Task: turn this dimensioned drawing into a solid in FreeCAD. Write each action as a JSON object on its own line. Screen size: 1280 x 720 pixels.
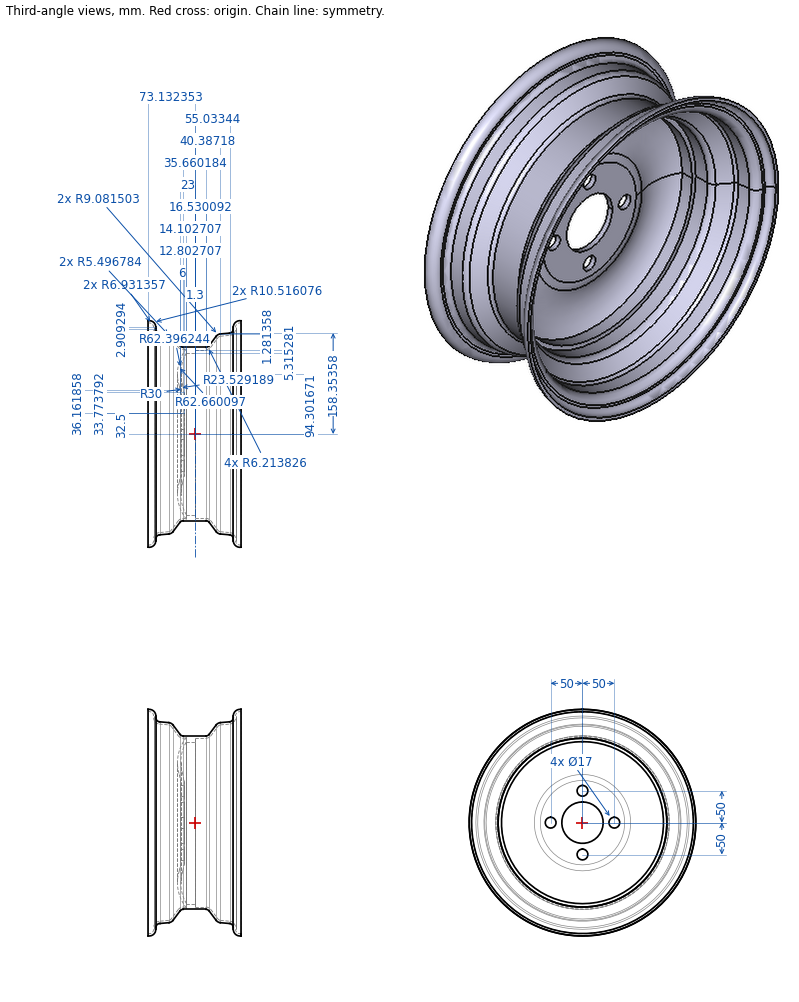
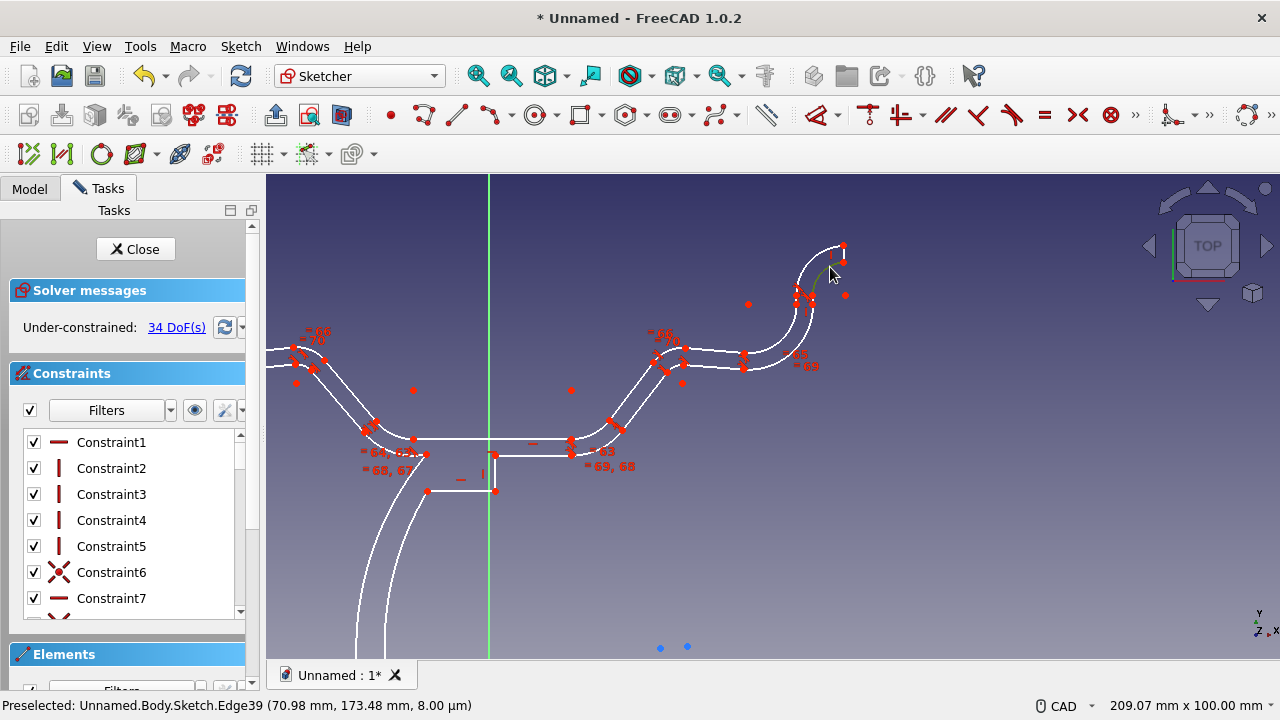
{"action": "key", "text": "e"}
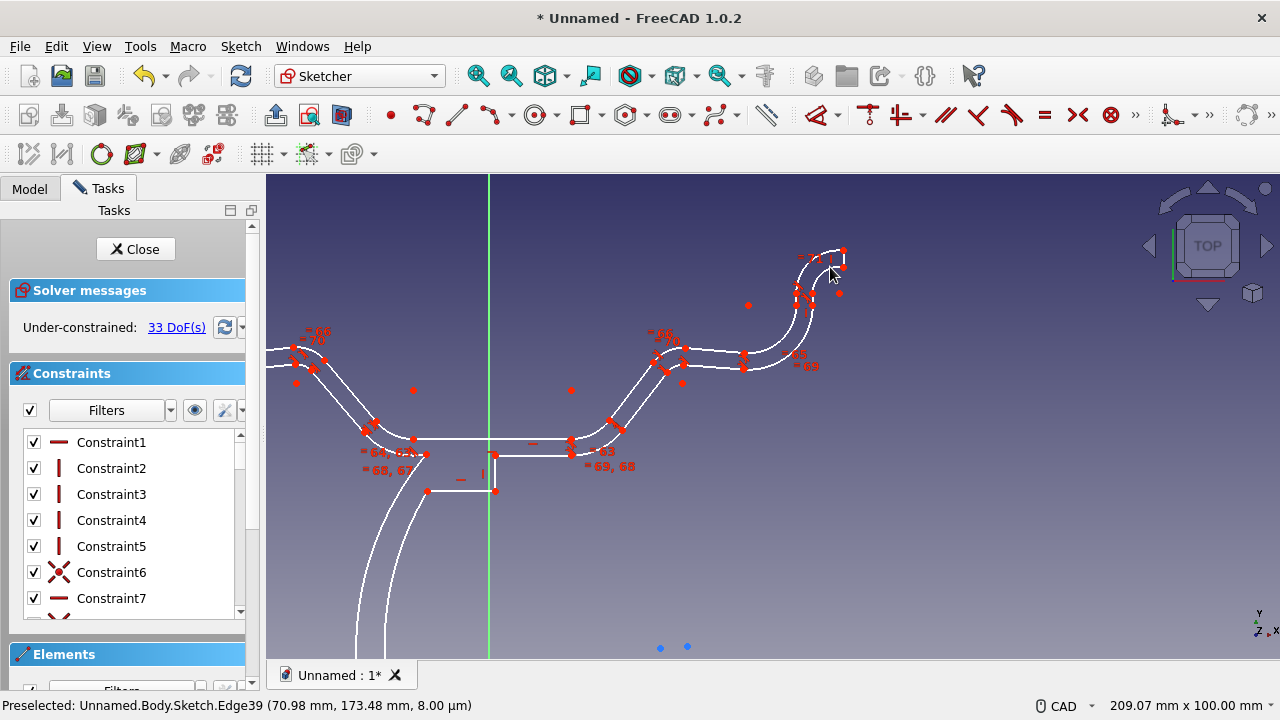
{"action": "left_click", "coordinate": [682, 384]}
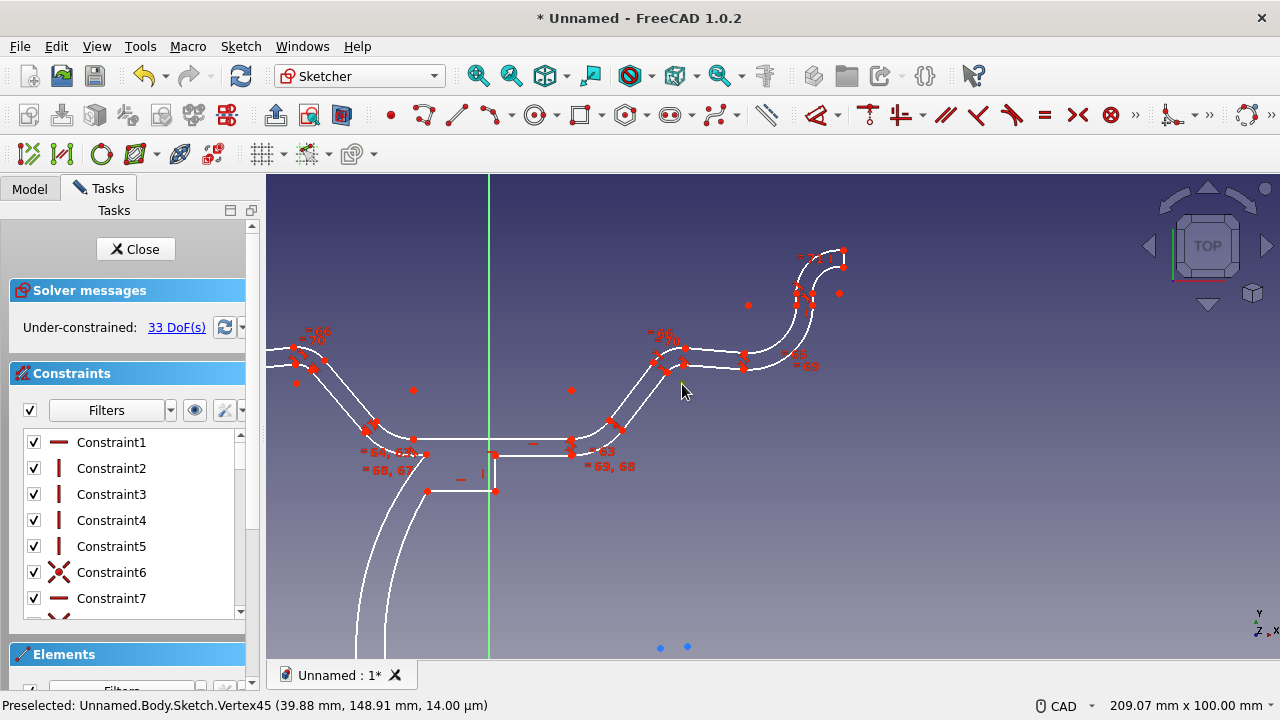
{"action": "left_click", "coordinate": [297, 383]}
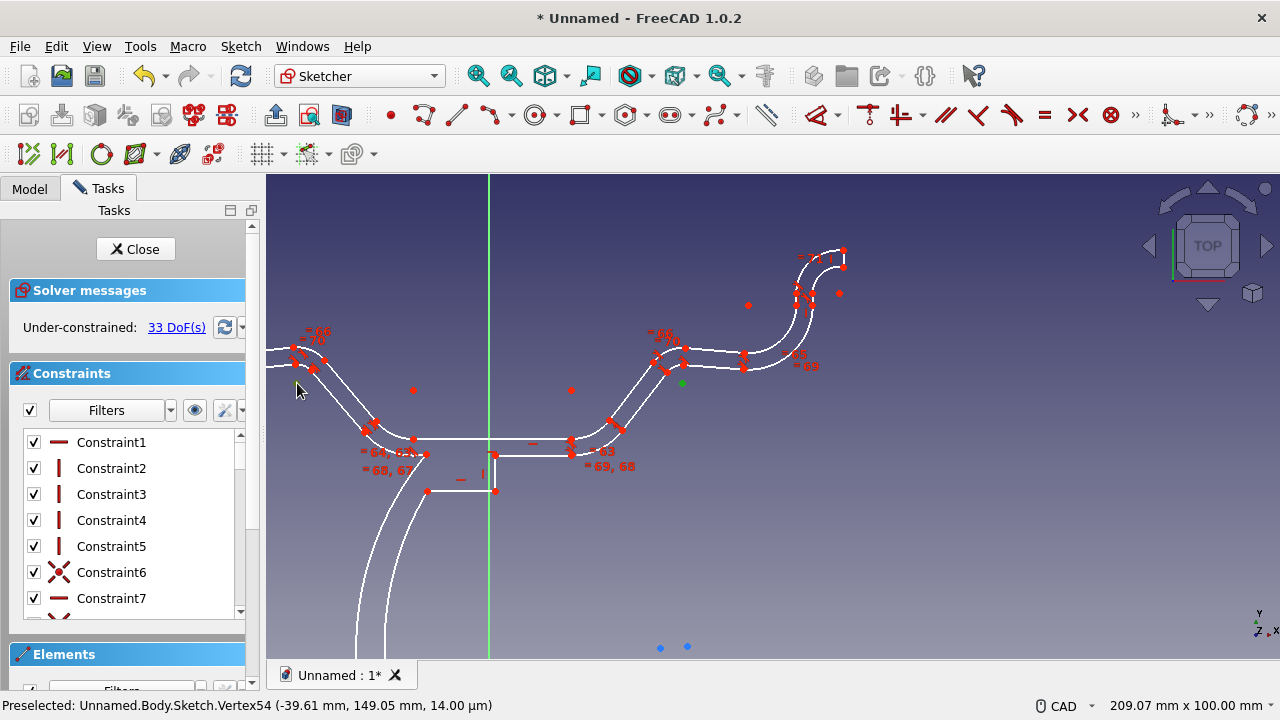
{"action": "left_click", "coordinate": [489, 600]}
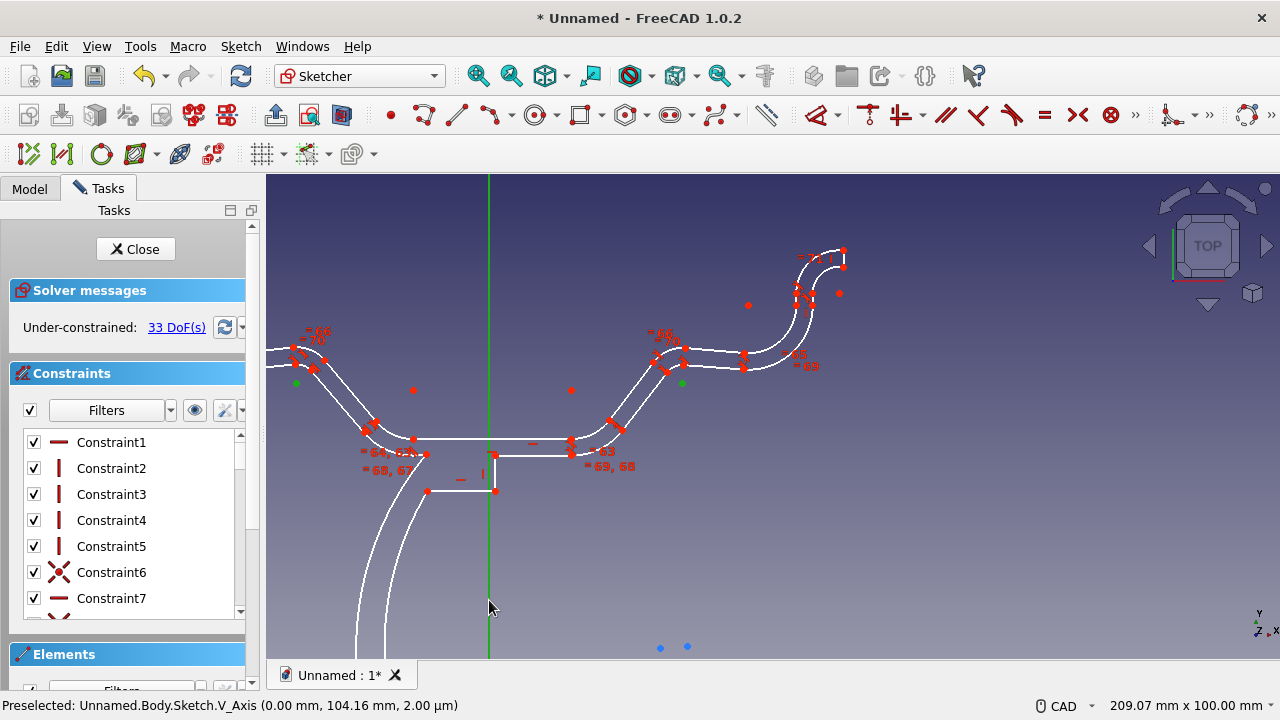
{"action": "left_click", "coordinate": [1078, 116]}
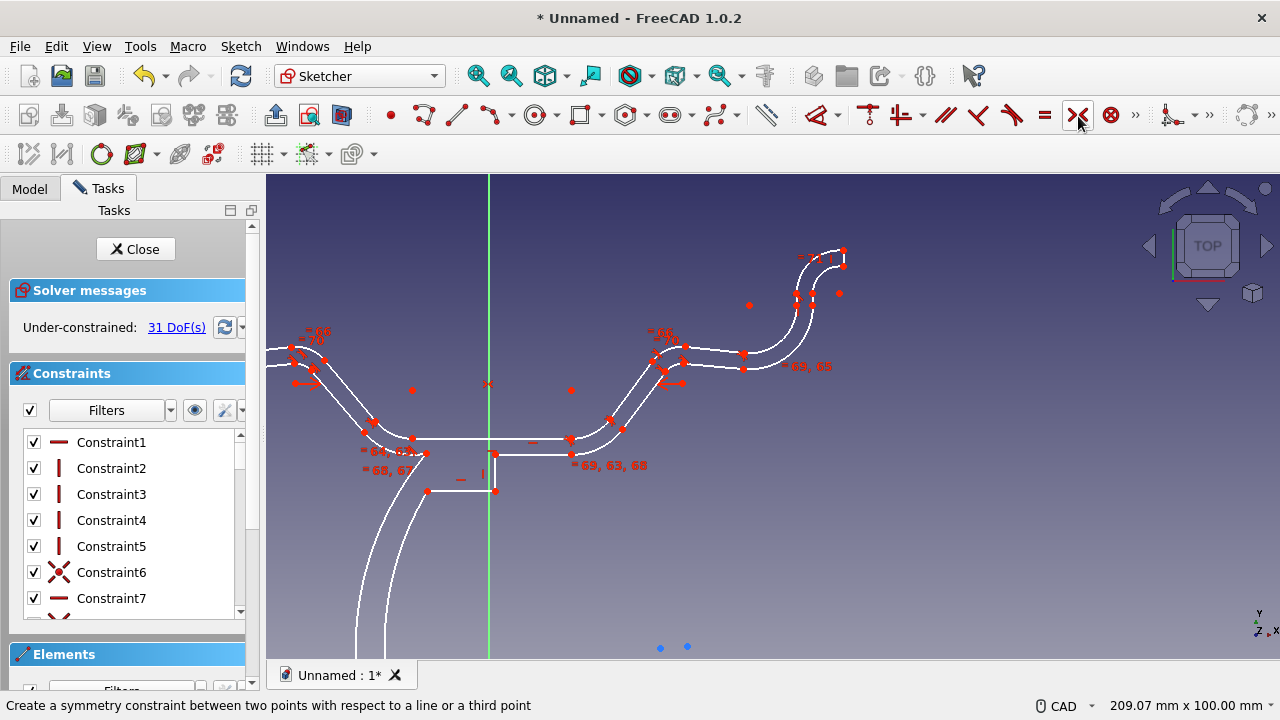
{"action": "scroll", "coordinate": [830, 266], "scroll_direction": "down", "scroll_amount": 5}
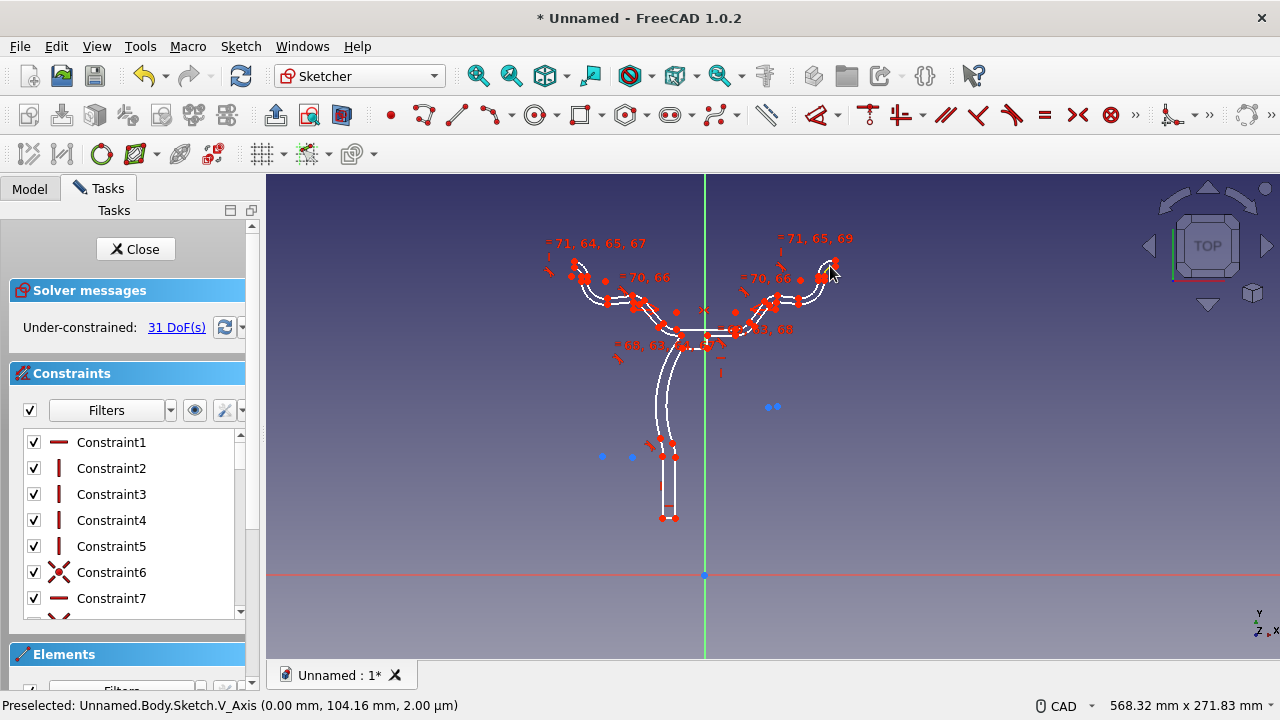
{"action": "left_click", "coordinate": [605, 281]}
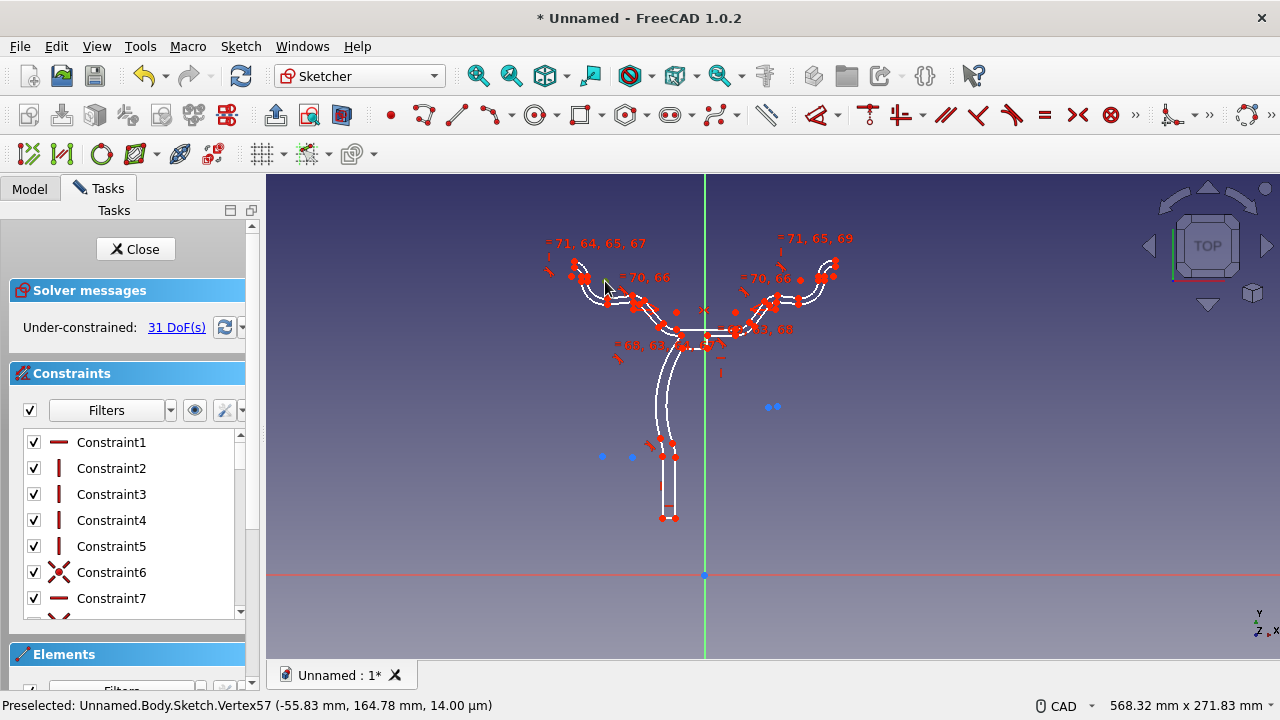
{"action": "left_click", "coordinate": [801, 281]}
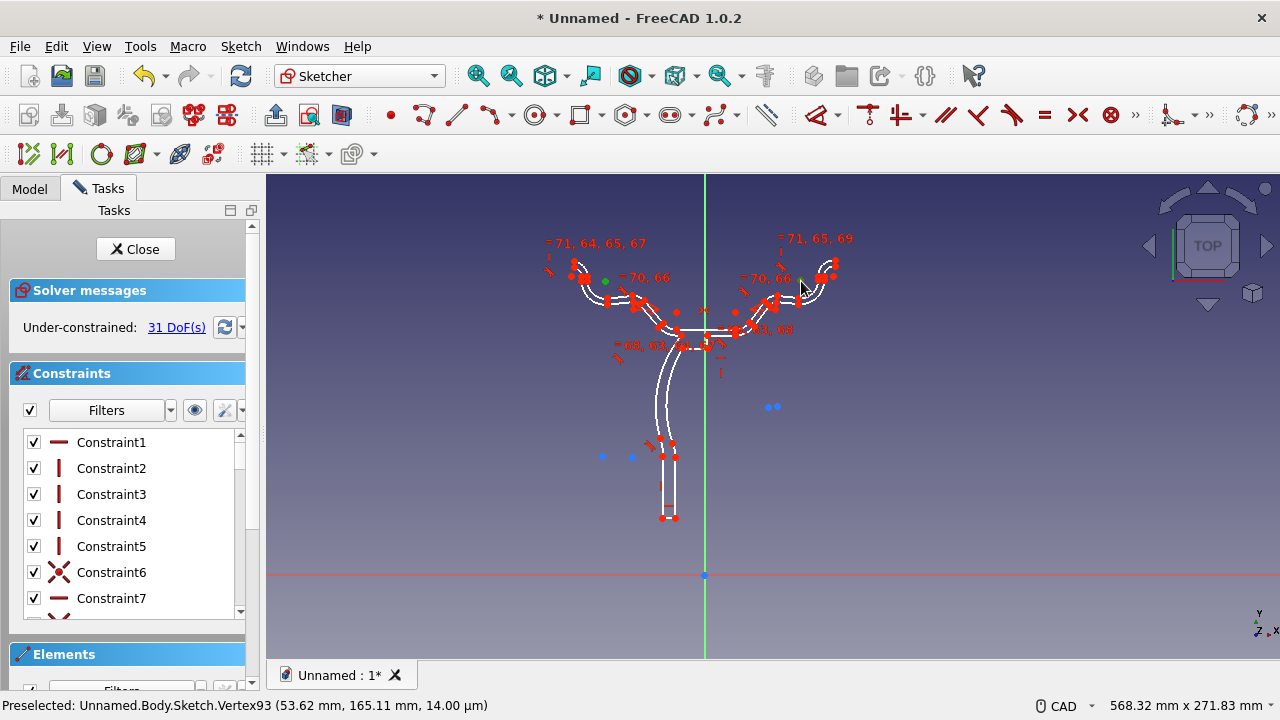
{"action": "left_click", "coordinate": [705, 539]}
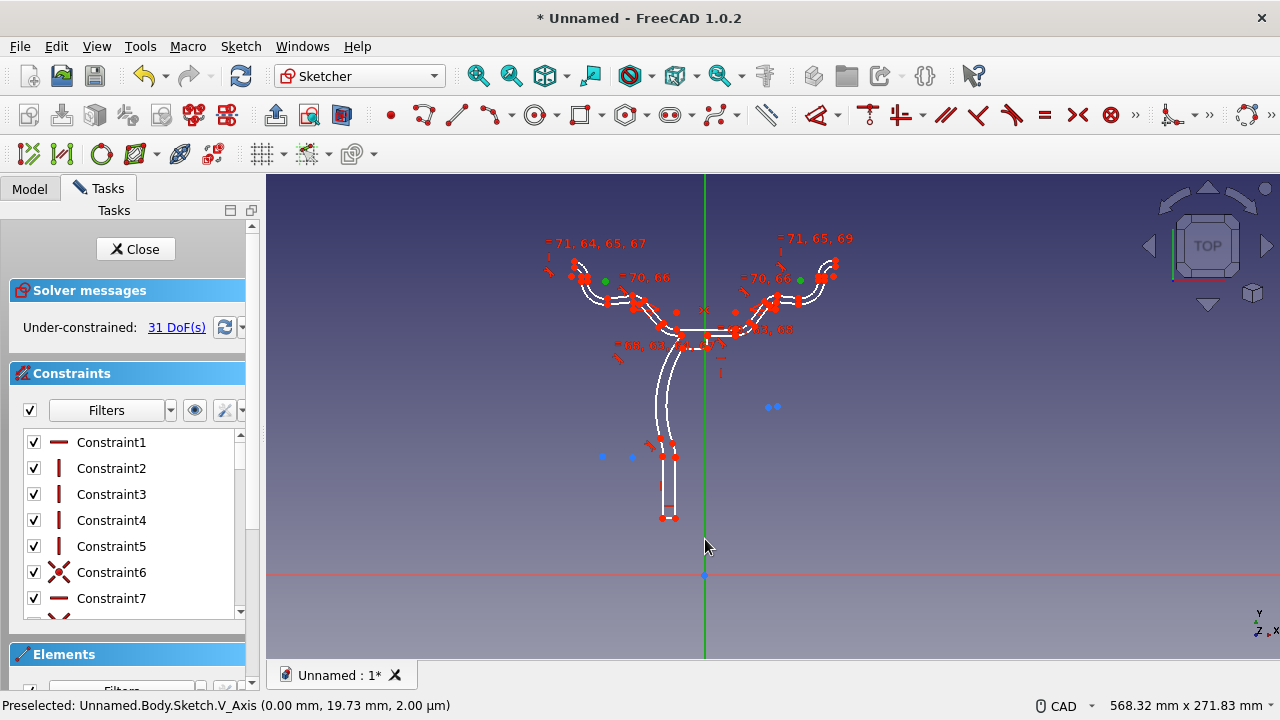
{"action": "key", "text": "s"}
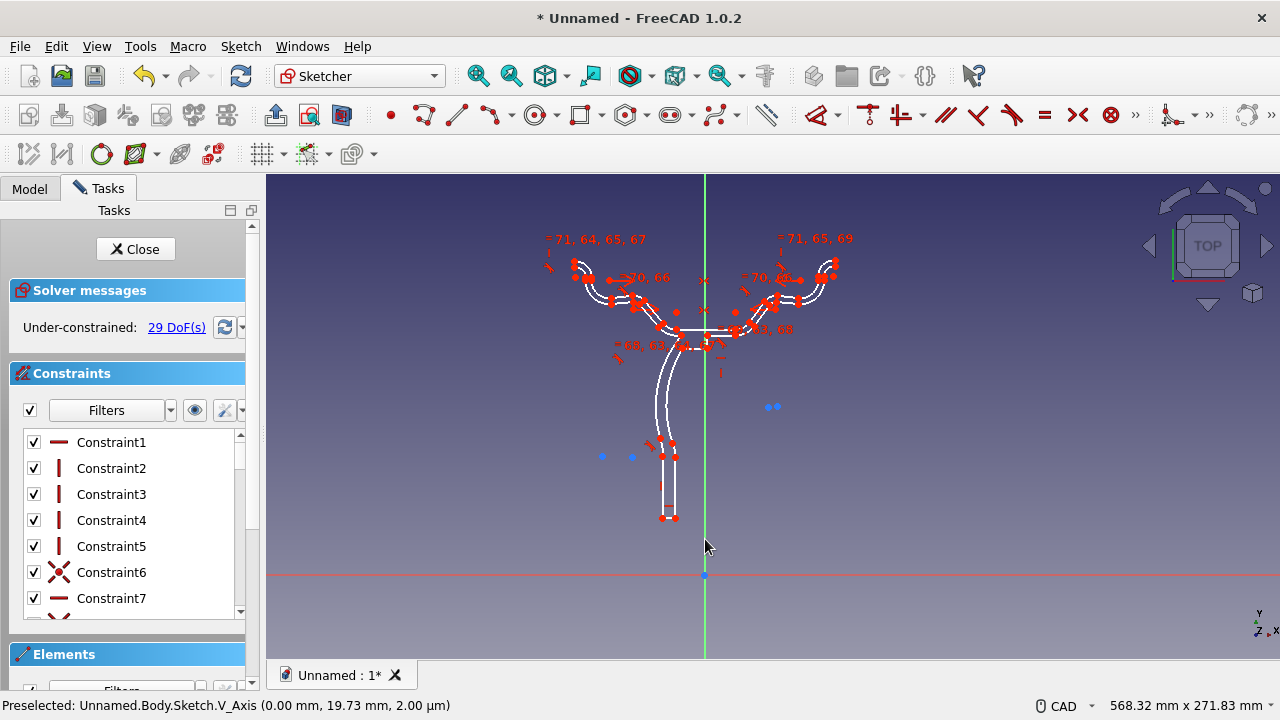
{"action": "scroll", "coordinate": [574, 268], "scroll_direction": "up", "scroll_amount": 4}